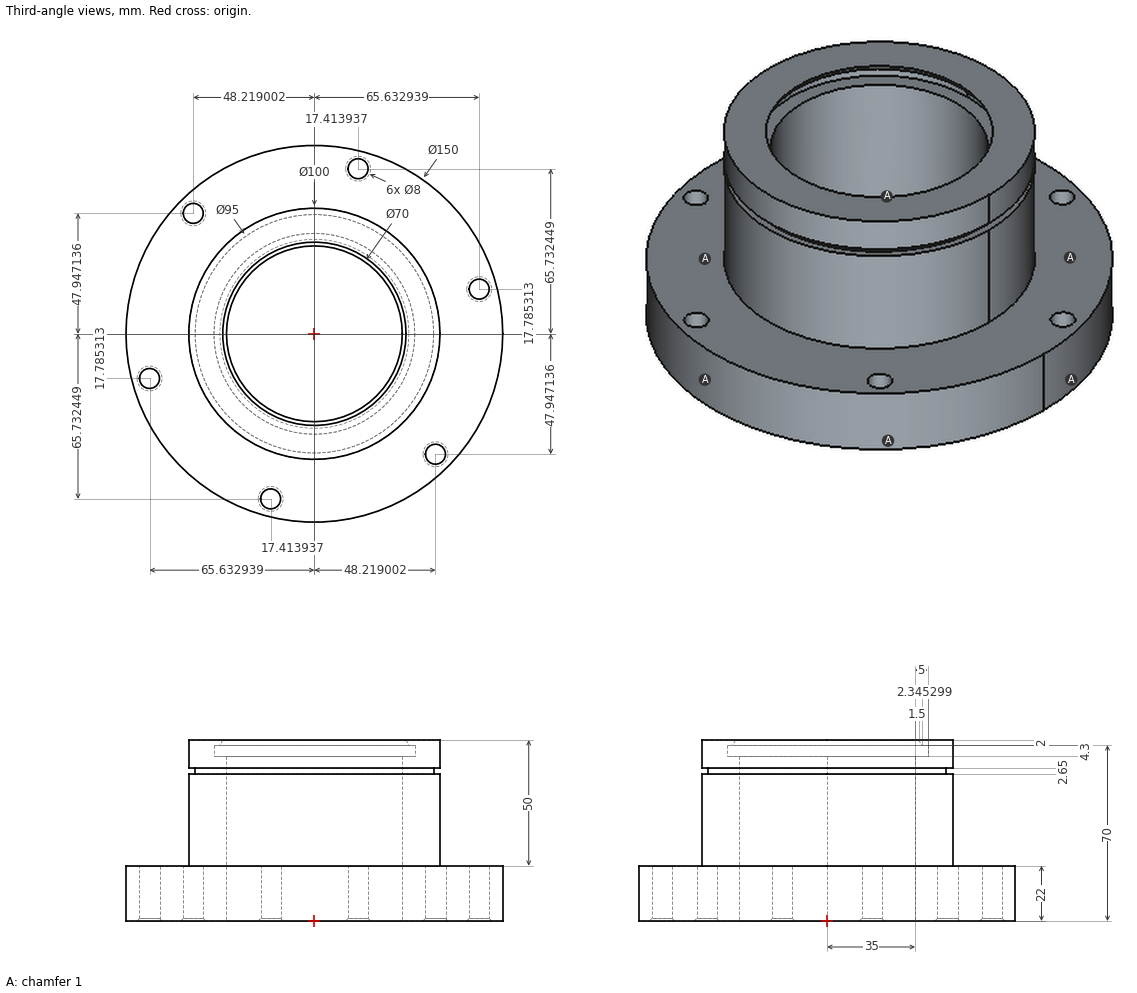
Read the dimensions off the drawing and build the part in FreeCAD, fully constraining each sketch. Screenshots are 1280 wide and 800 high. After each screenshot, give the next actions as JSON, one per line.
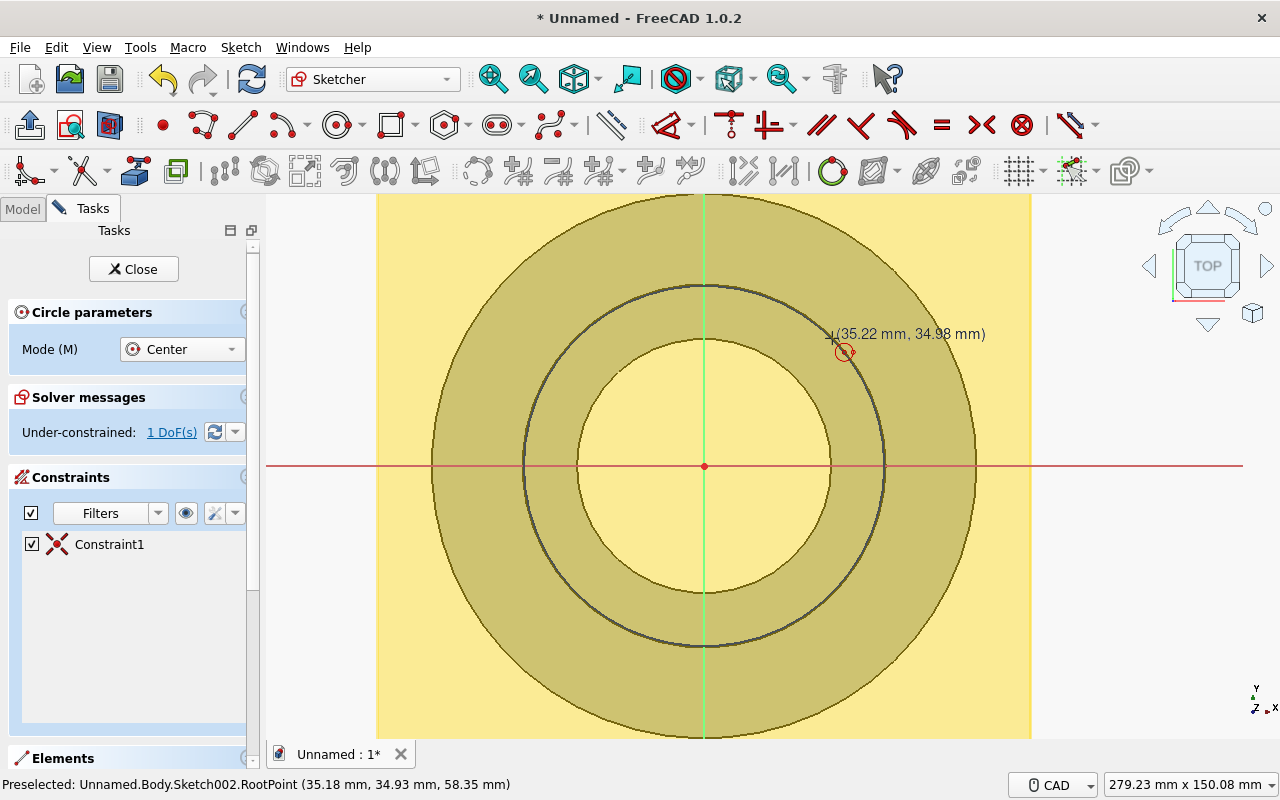
{"action": "left_click", "coordinate": [704, 466]}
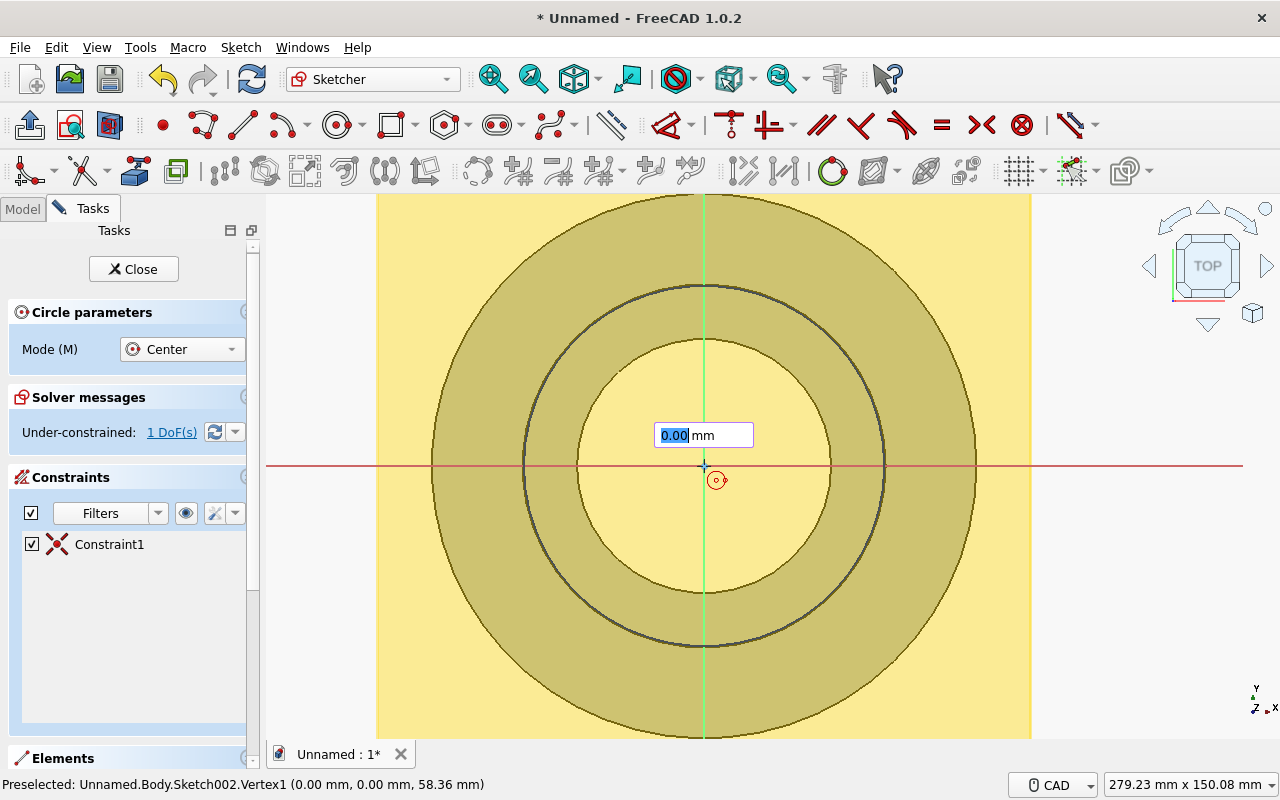
{"action": "scroll", "coordinate": [826, 344], "scroll_direction": "up", "scroll_amount": 3}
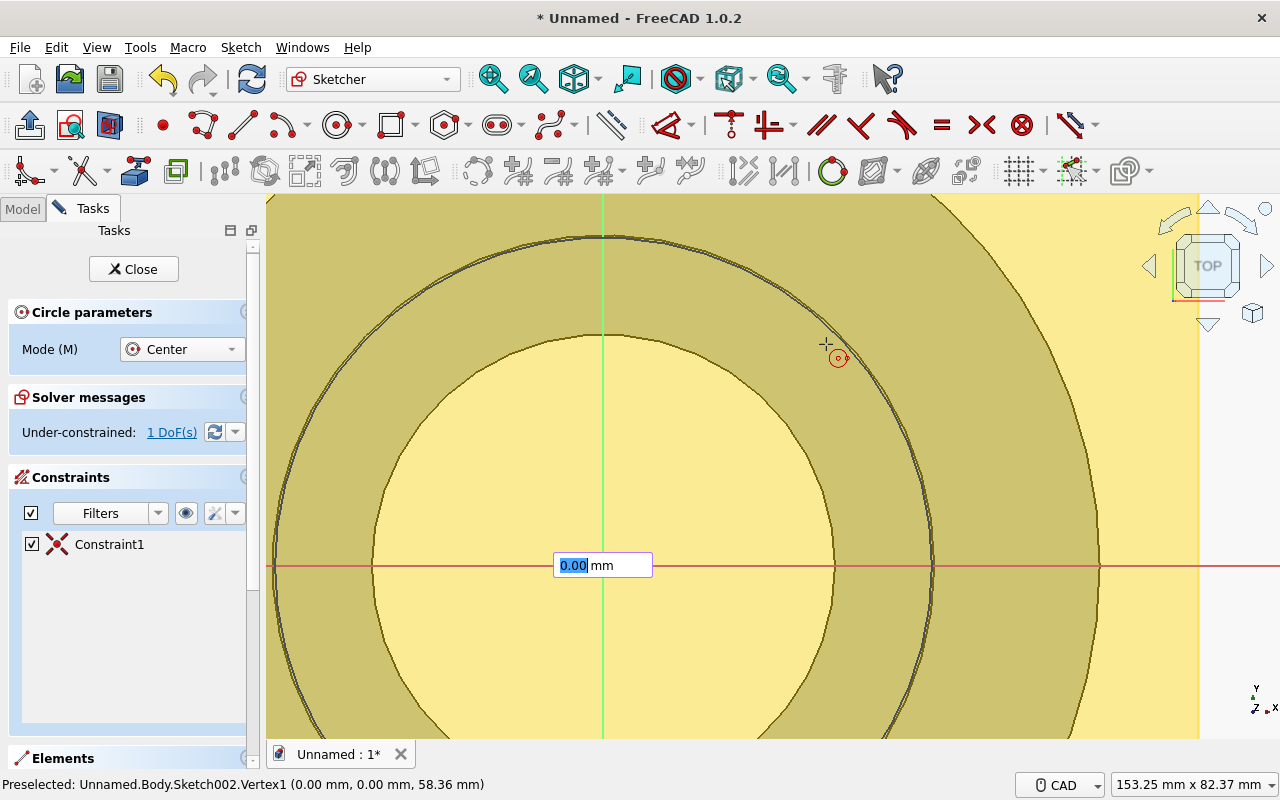
{"action": "left_click", "coordinate": [826, 344]}
{"action": "key", "text": "Escape"}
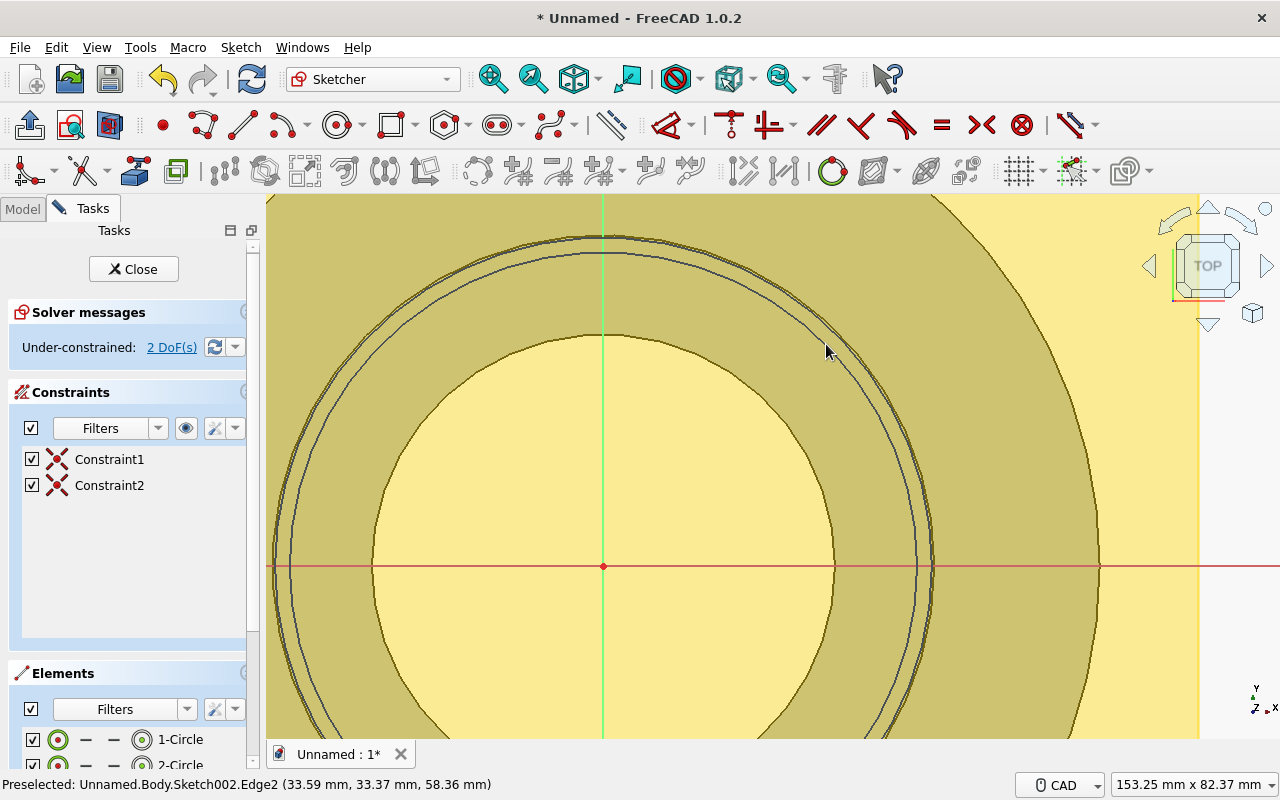
{"action": "left_click", "coordinate": [666, 126]}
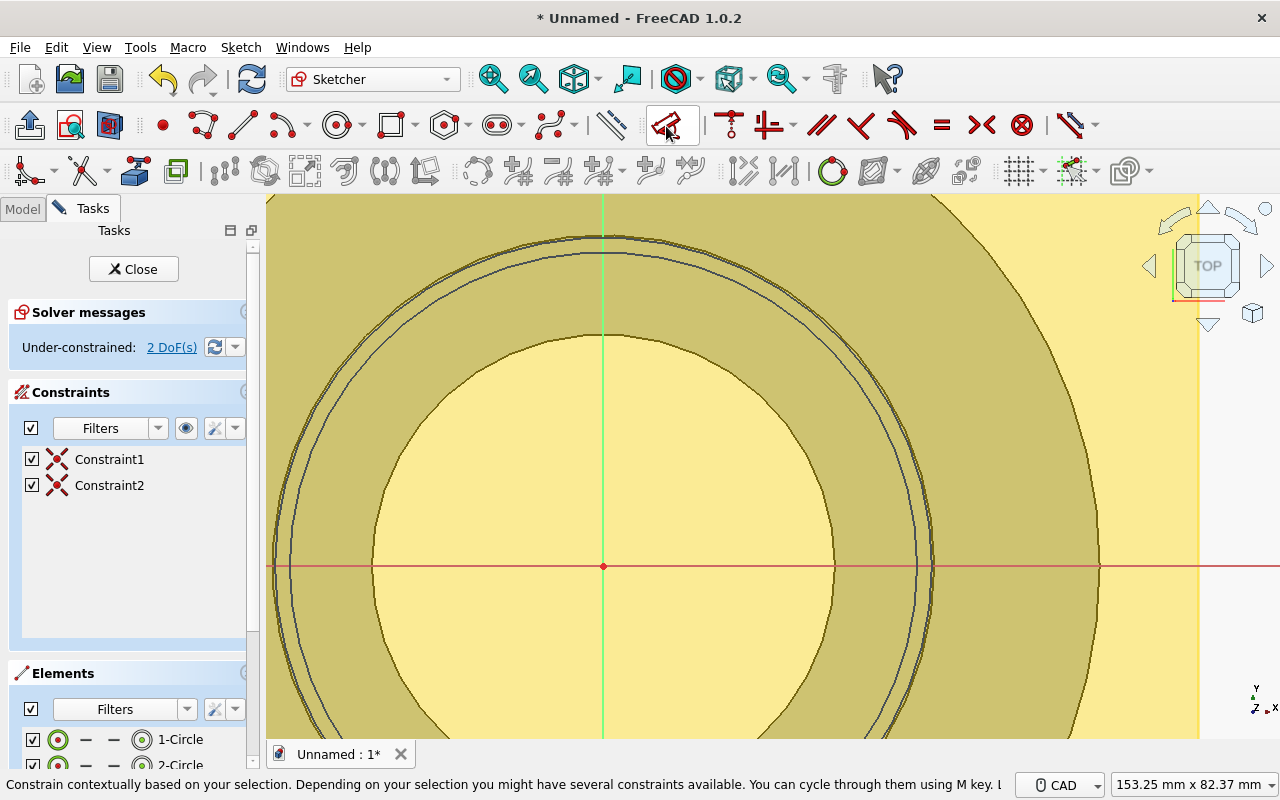
{"action": "left_click", "coordinate": [835, 333]}
{"action": "left_click", "coordinate": [858, 310]}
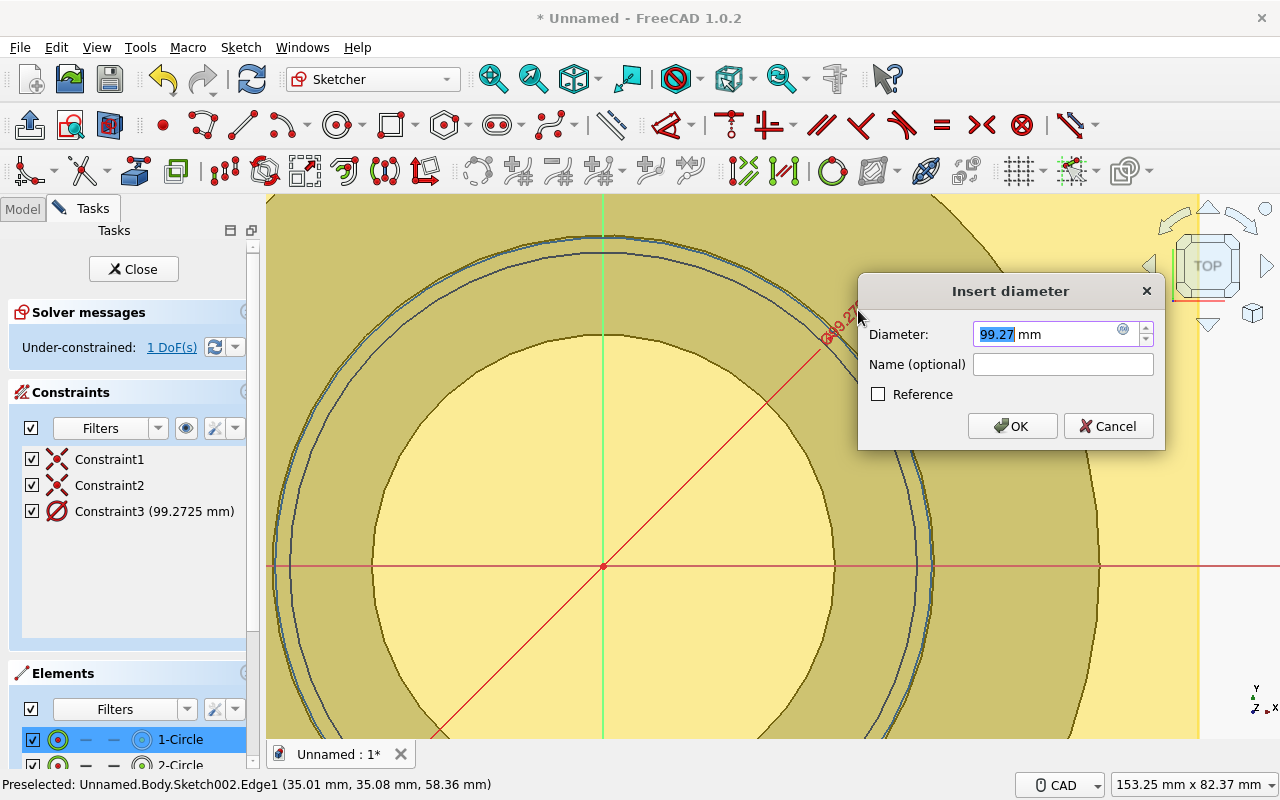
{"action": "type", "text": "100"}
{"action": "key", "text": "Return"}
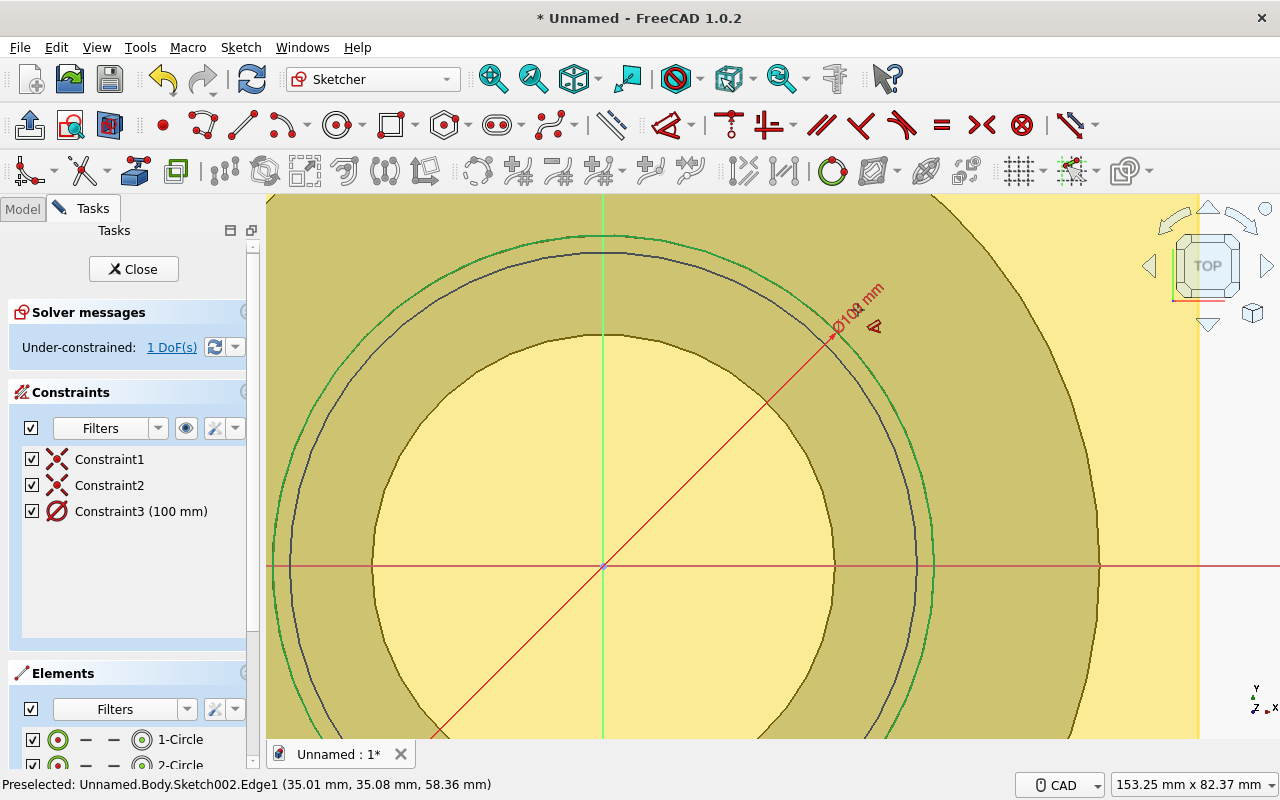
{"action": "left_click", "coordinate": [825, 344]}
{"action": "left_click", "coordinate": [935, 468]}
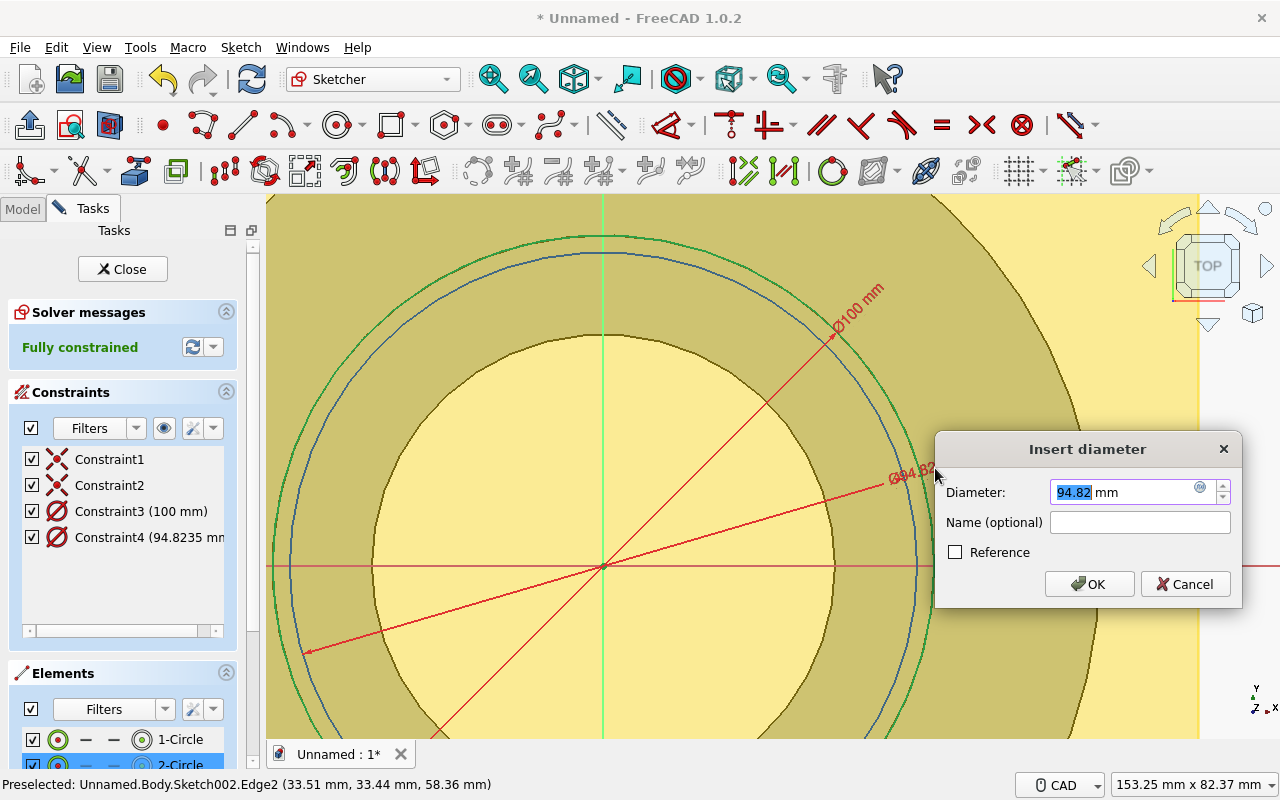
{"action": "type", "text": "95"}
{"action": "key", "text": "Return"}
{"action": "key", "text": "Escape"}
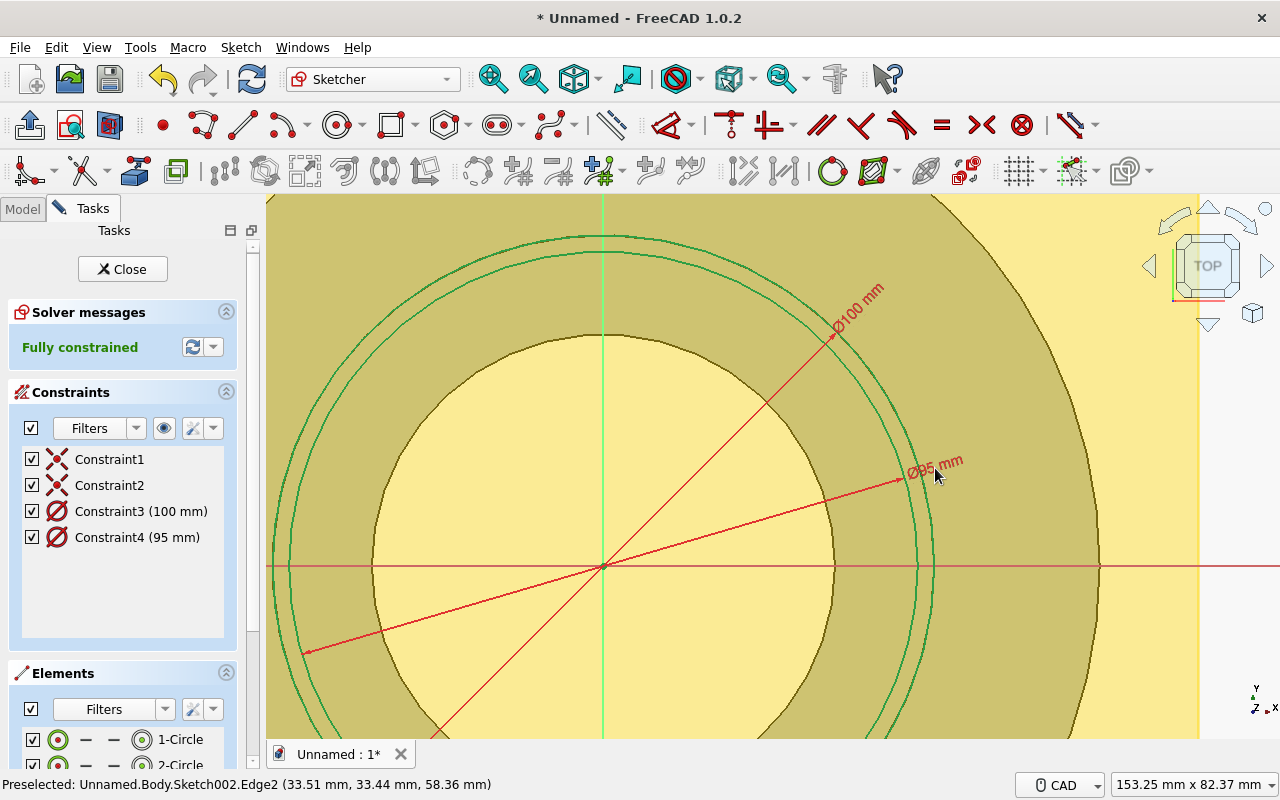
{"action": "left_click", "coordinate": [123, 269]}